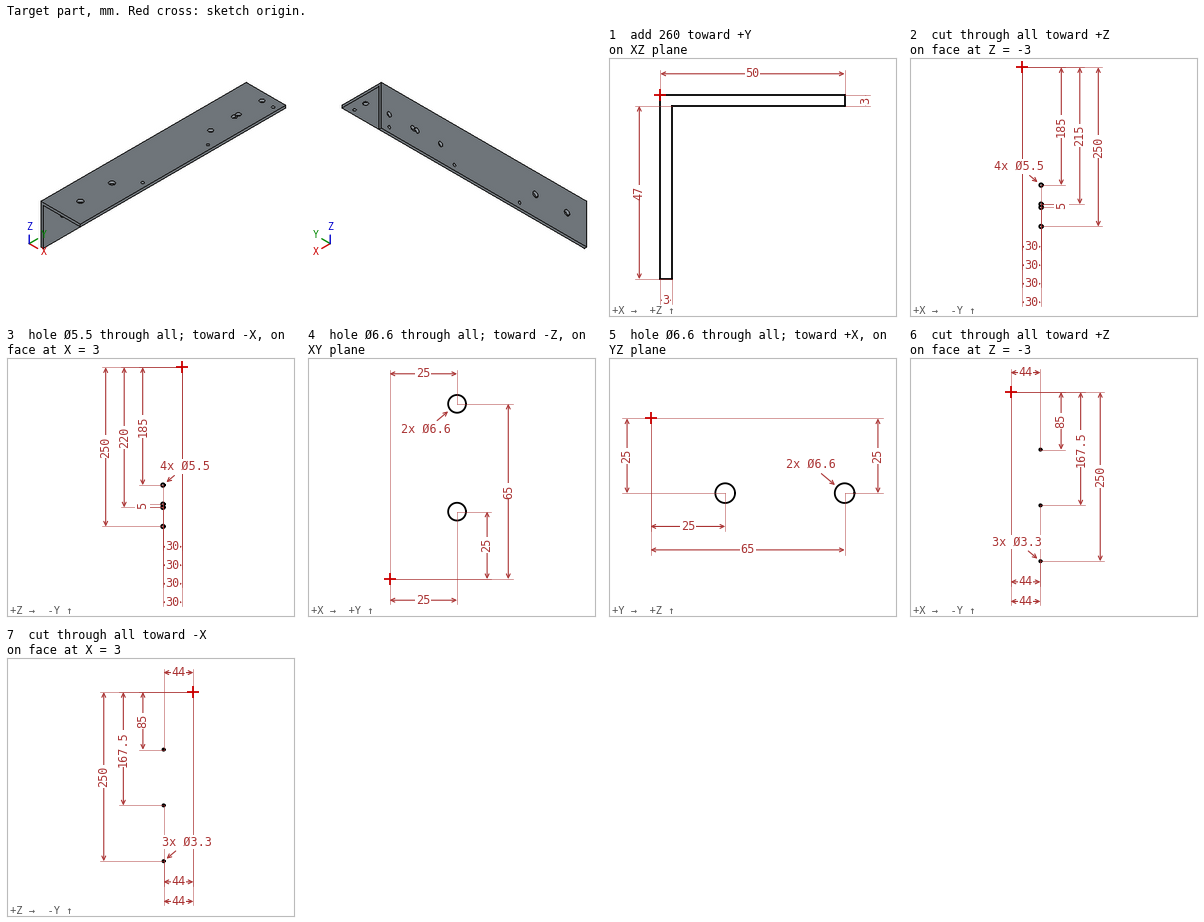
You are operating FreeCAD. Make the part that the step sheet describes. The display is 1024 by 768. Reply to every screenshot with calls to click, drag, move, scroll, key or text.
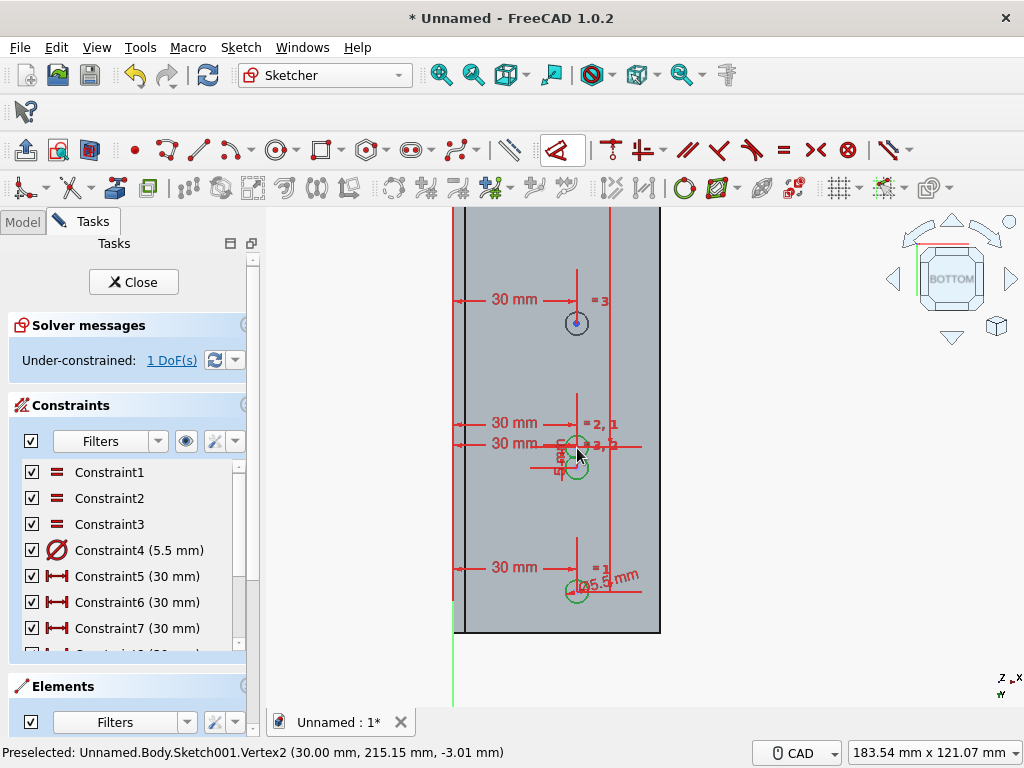
click(577, 324)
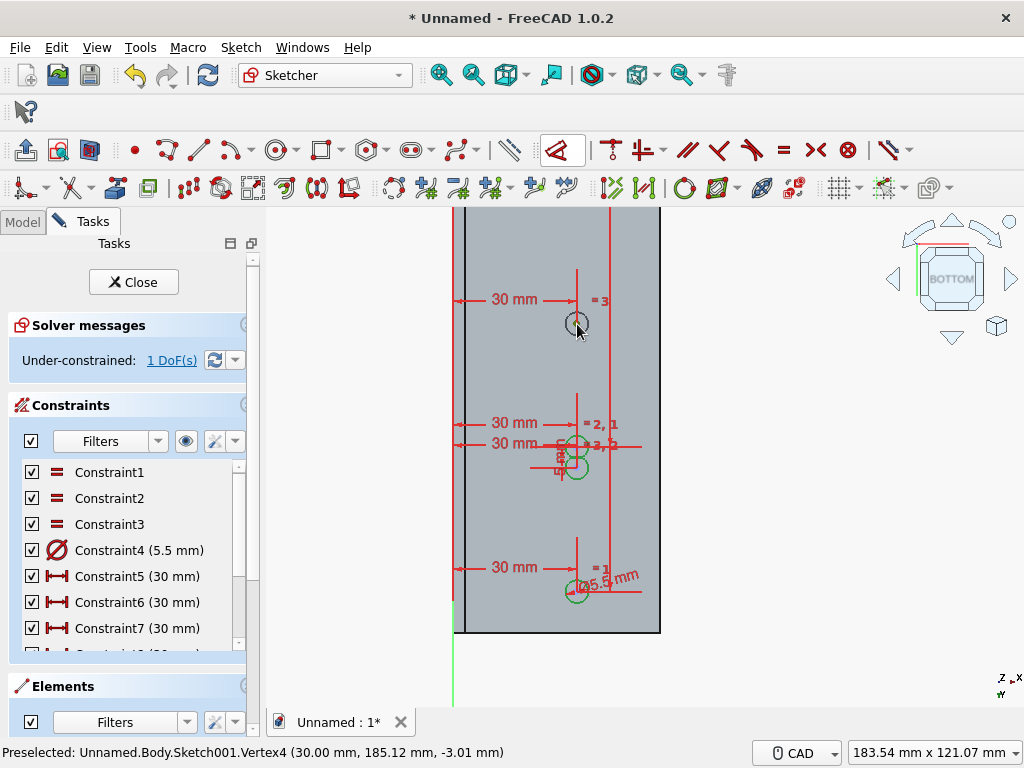
key(i)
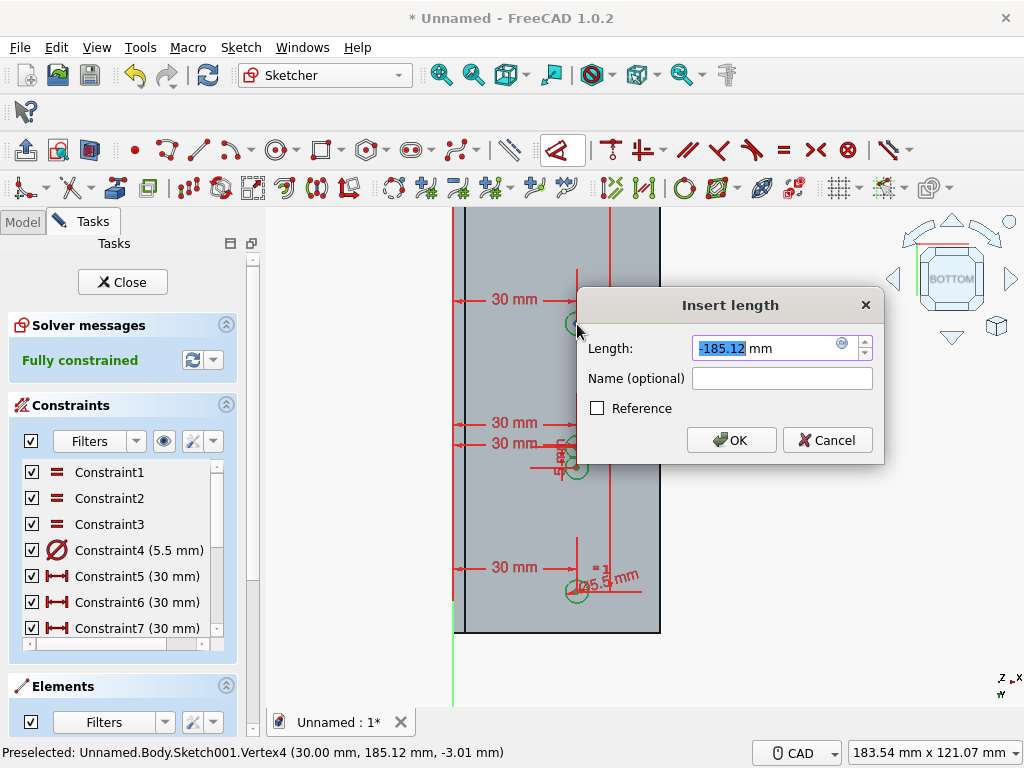
text(-185)
key(Return)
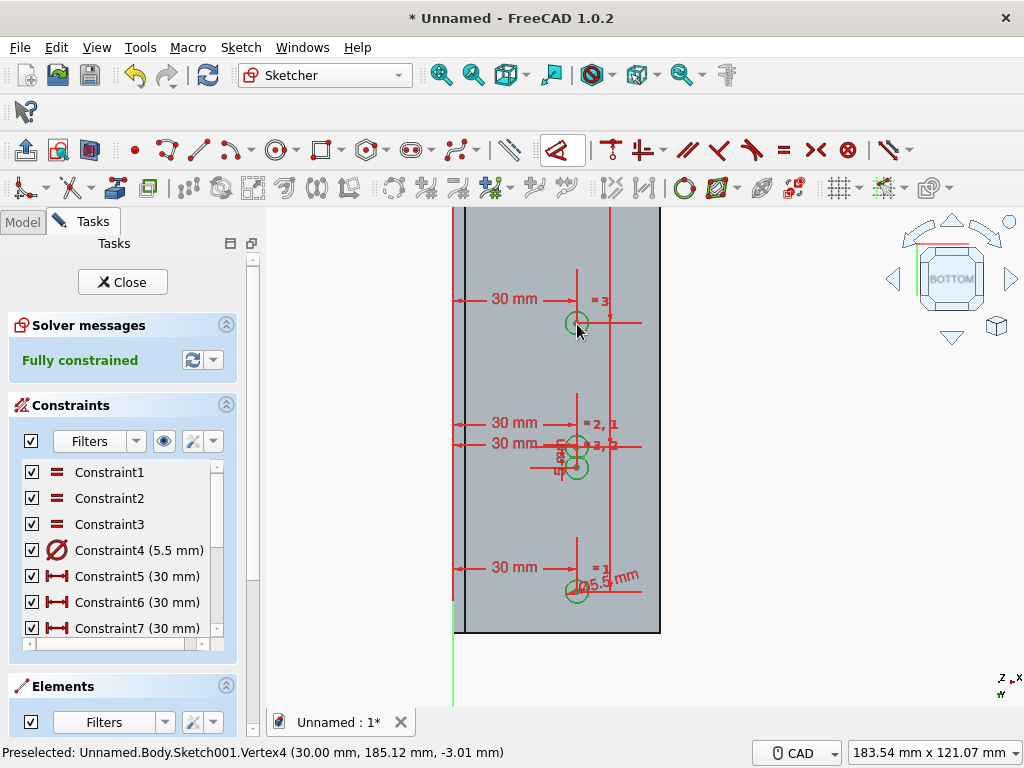
click(123, 282)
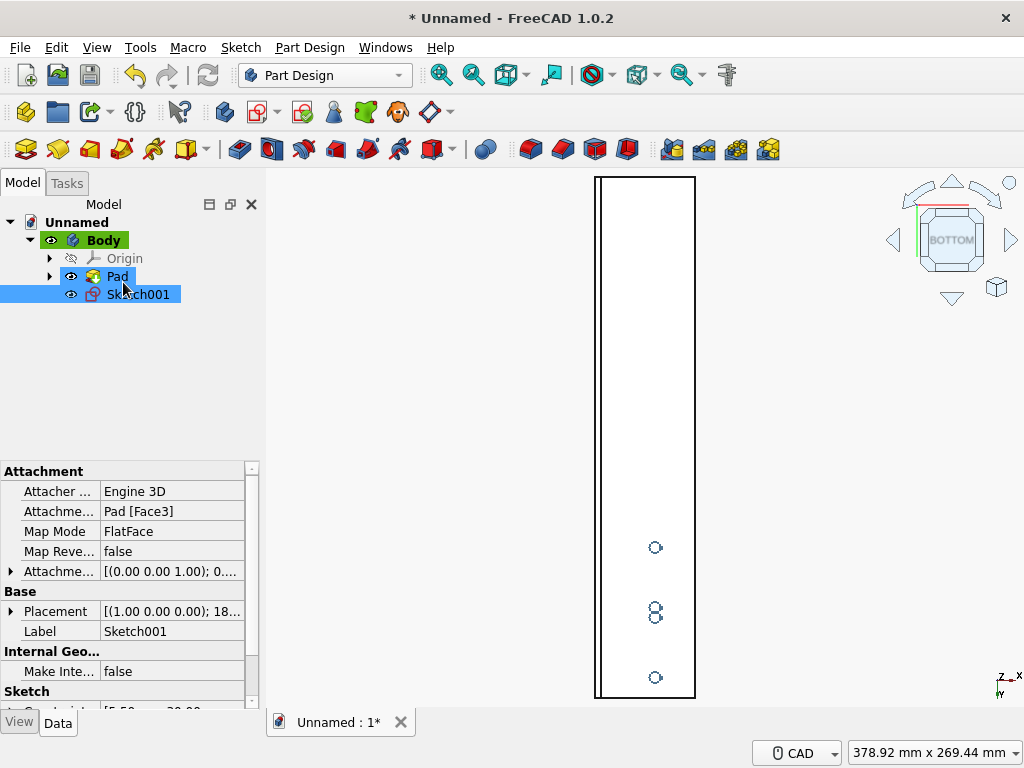
click(240, 150)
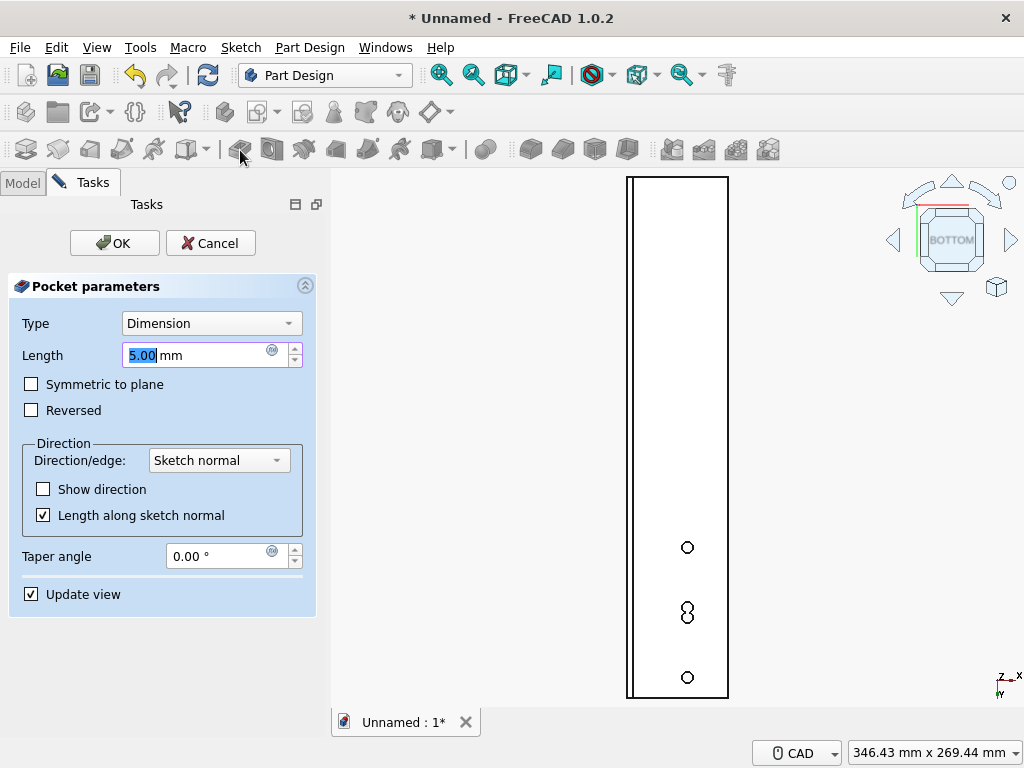
click(212, 324)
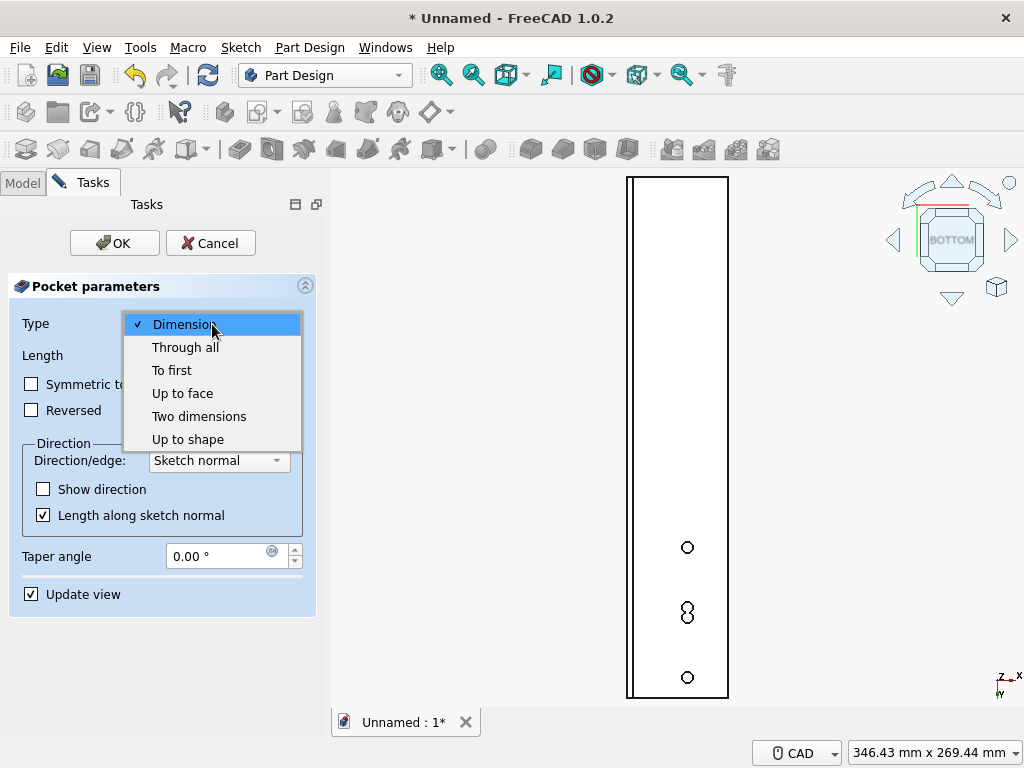
click(212, 348)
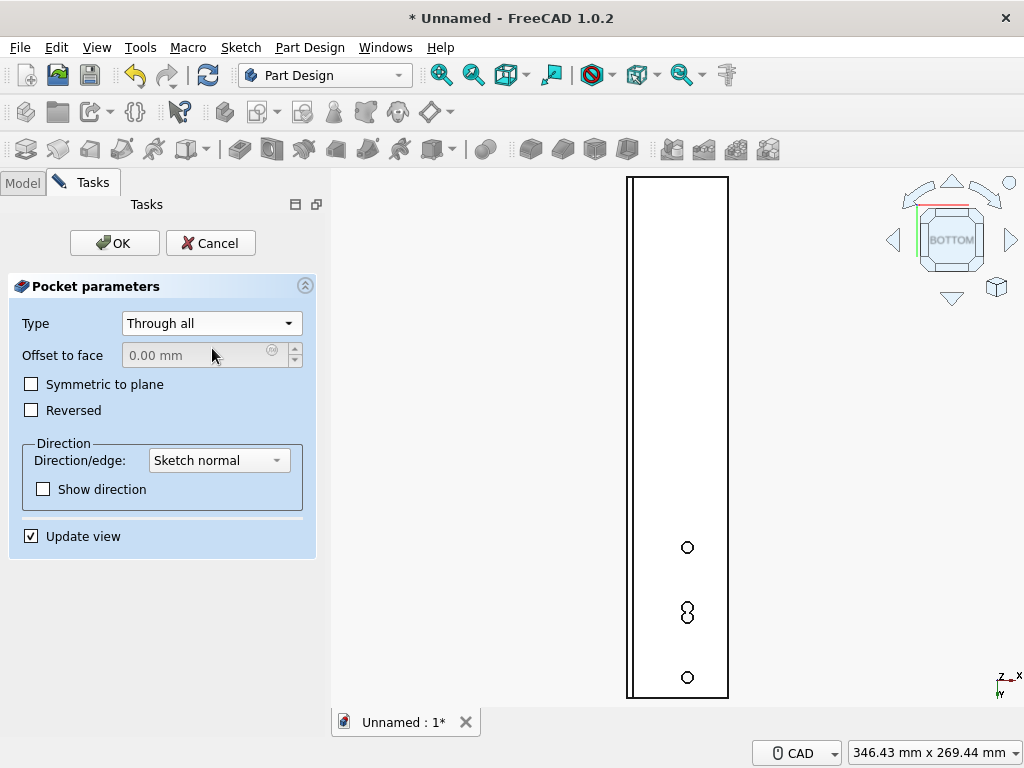
click(115, 243)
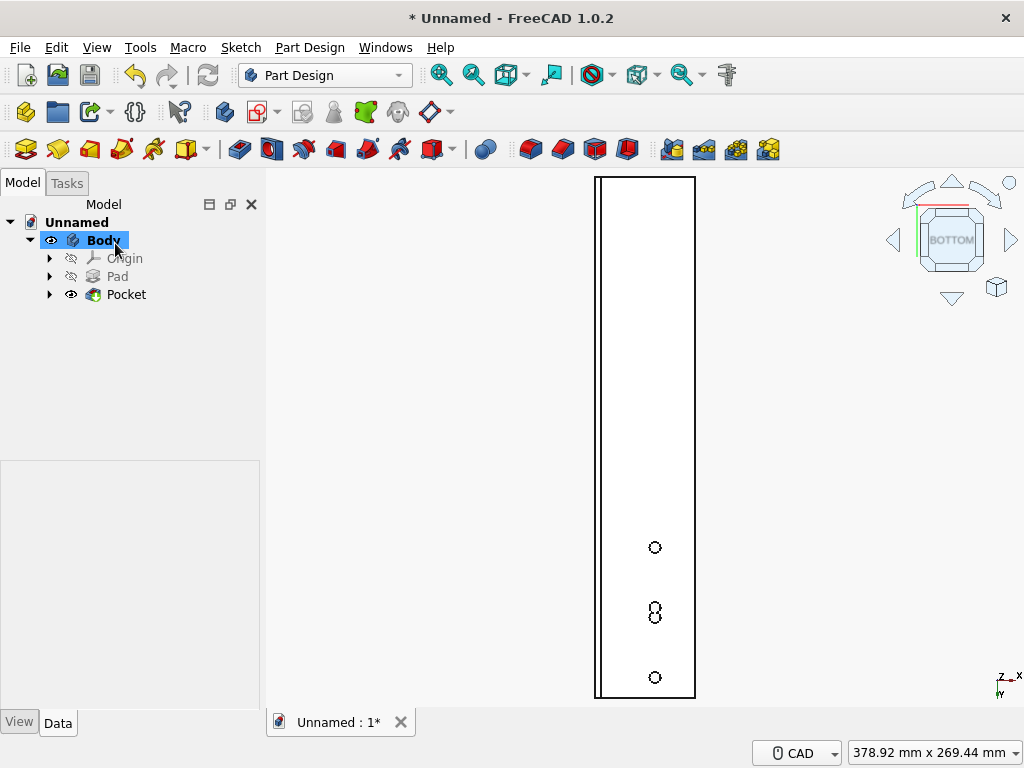
key(0)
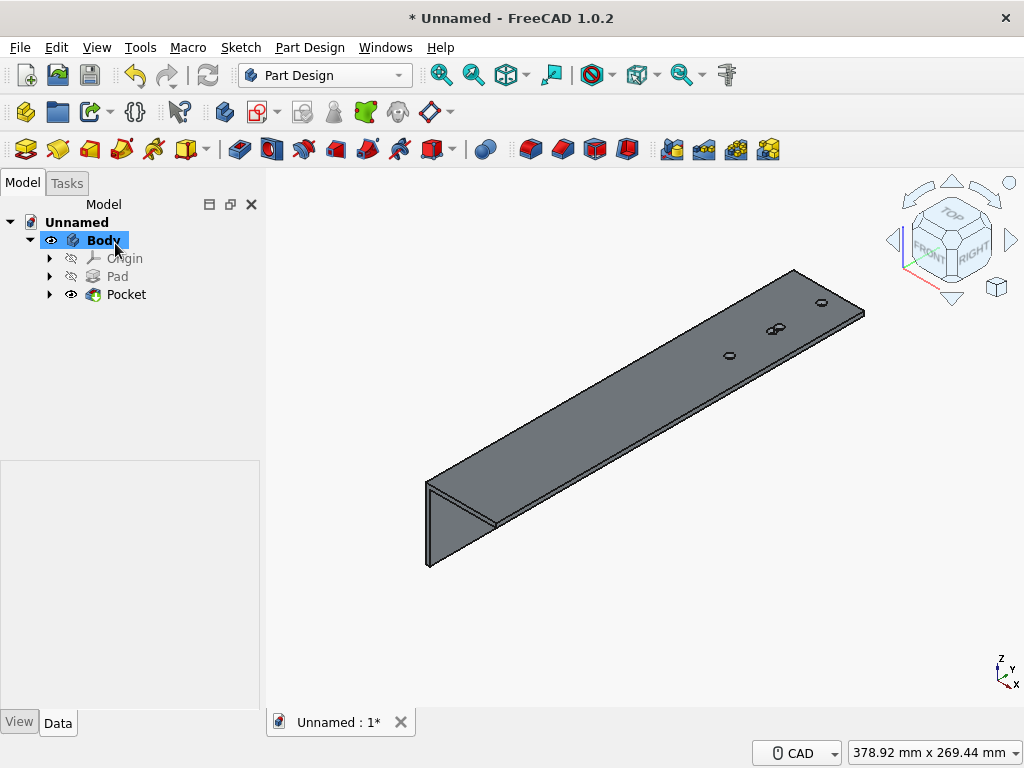
key(3)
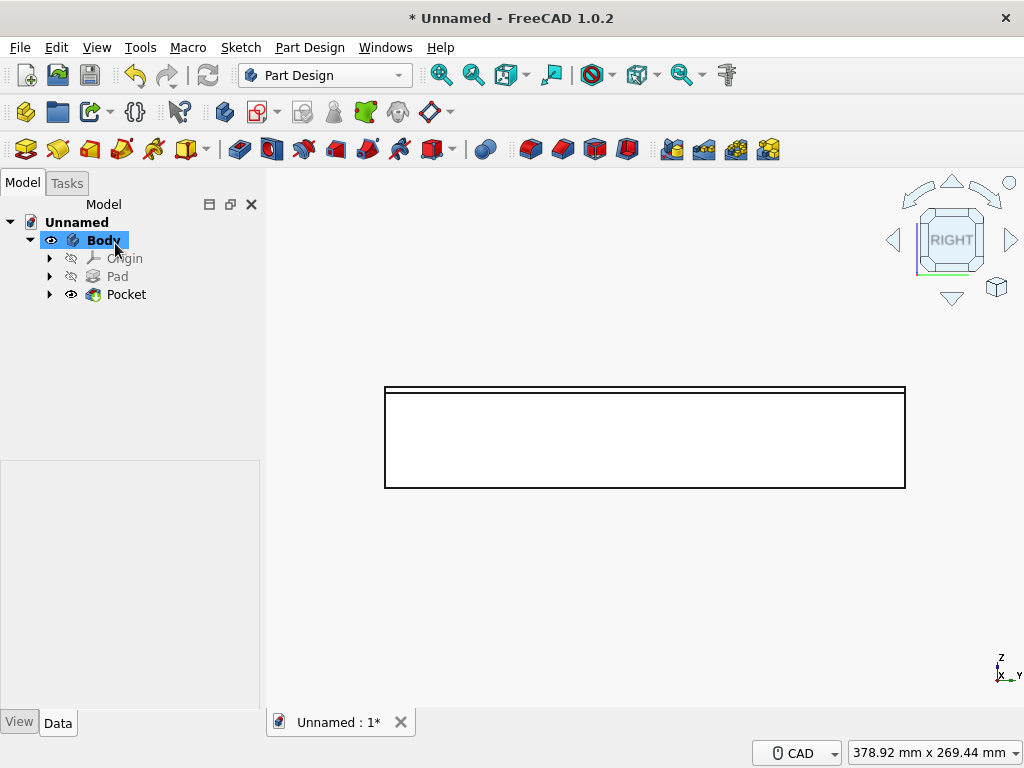
click(571, 440)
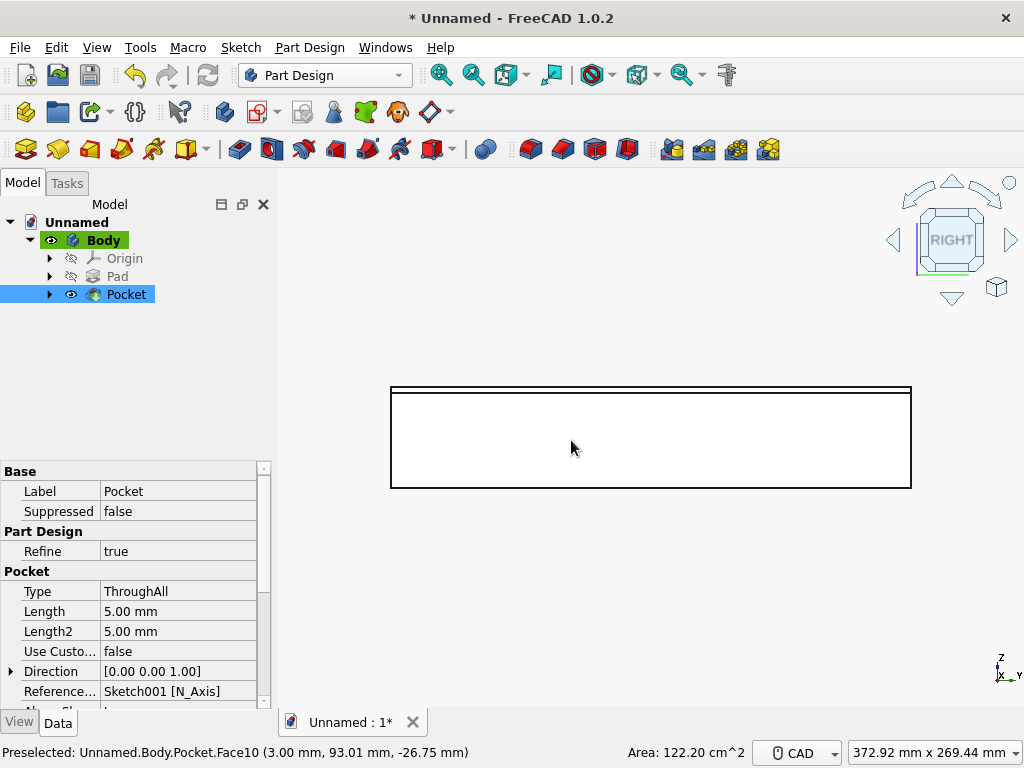
click(258, 112)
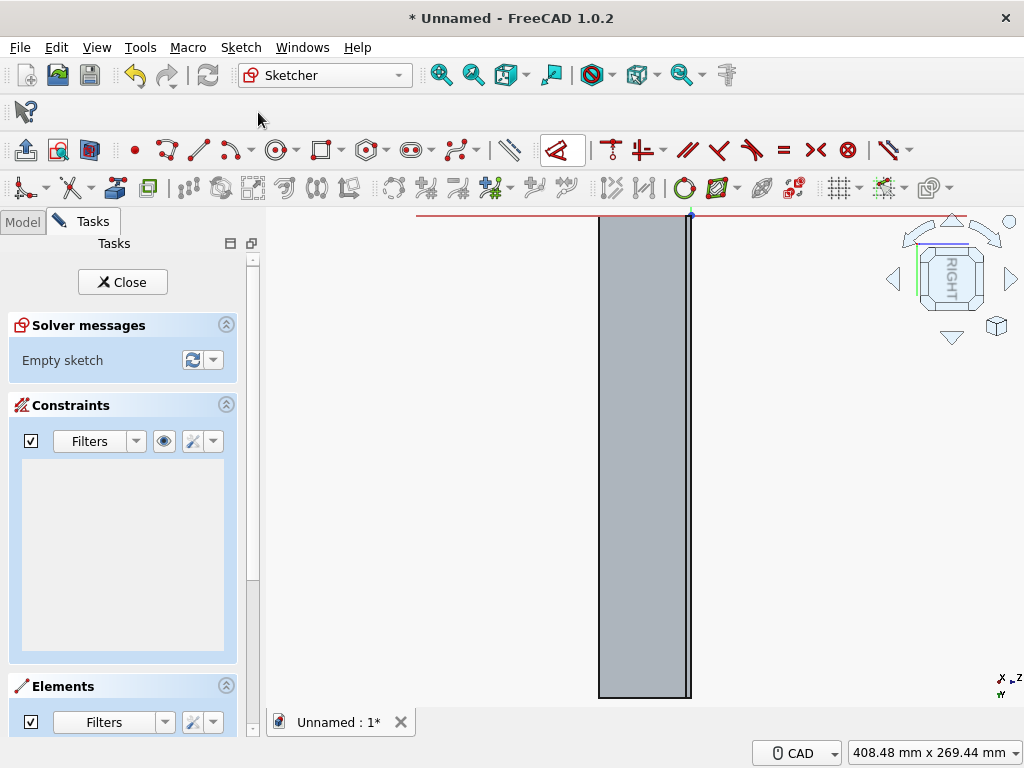
key(q)
key(s)